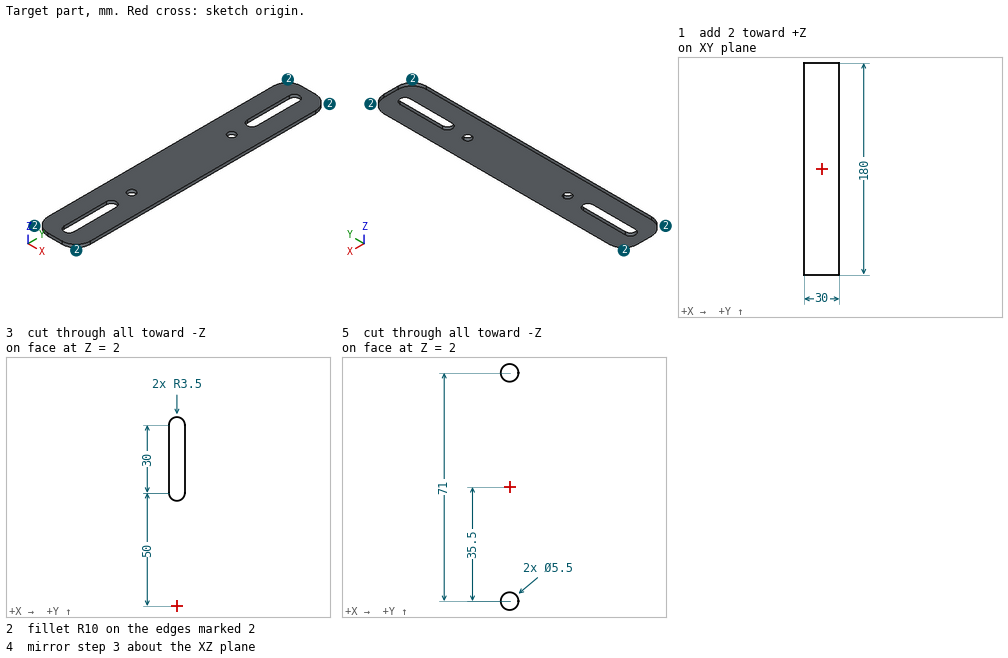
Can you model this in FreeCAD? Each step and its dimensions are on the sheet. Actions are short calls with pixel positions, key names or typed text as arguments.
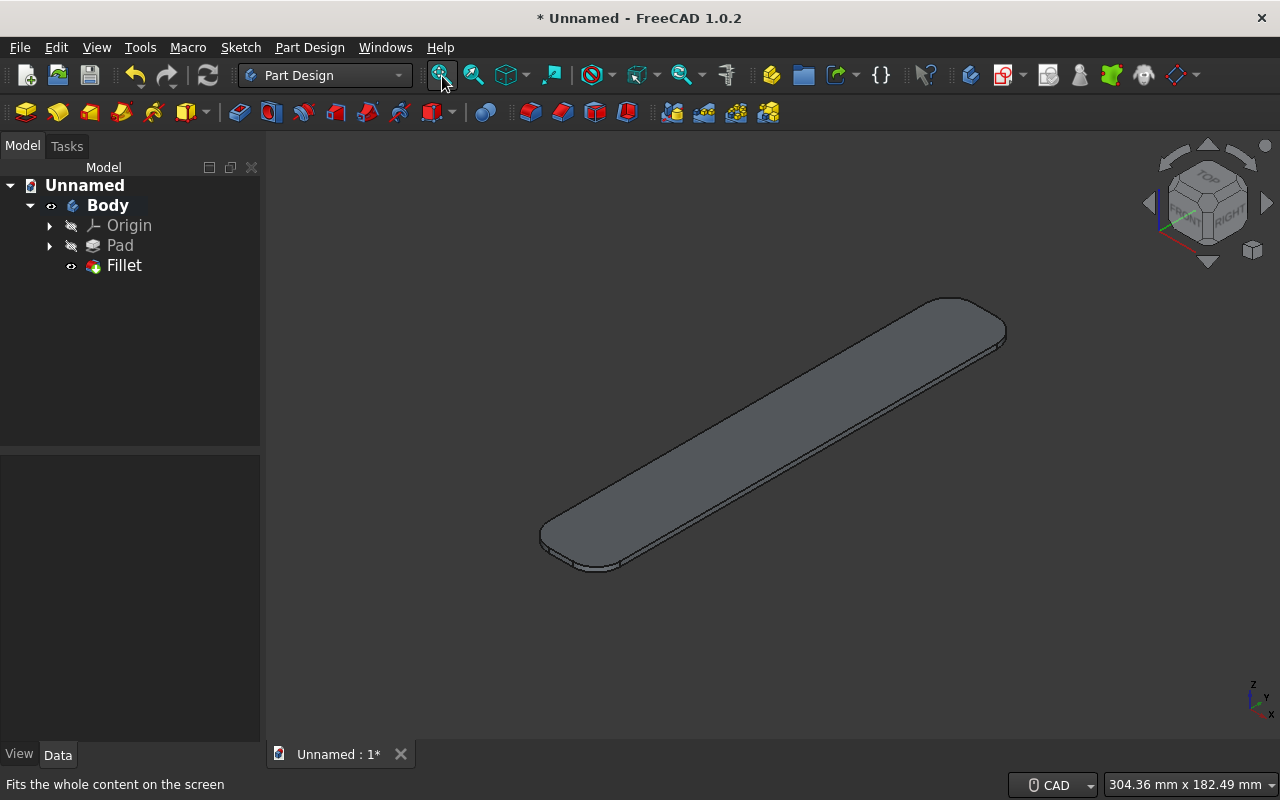
click(894, 361)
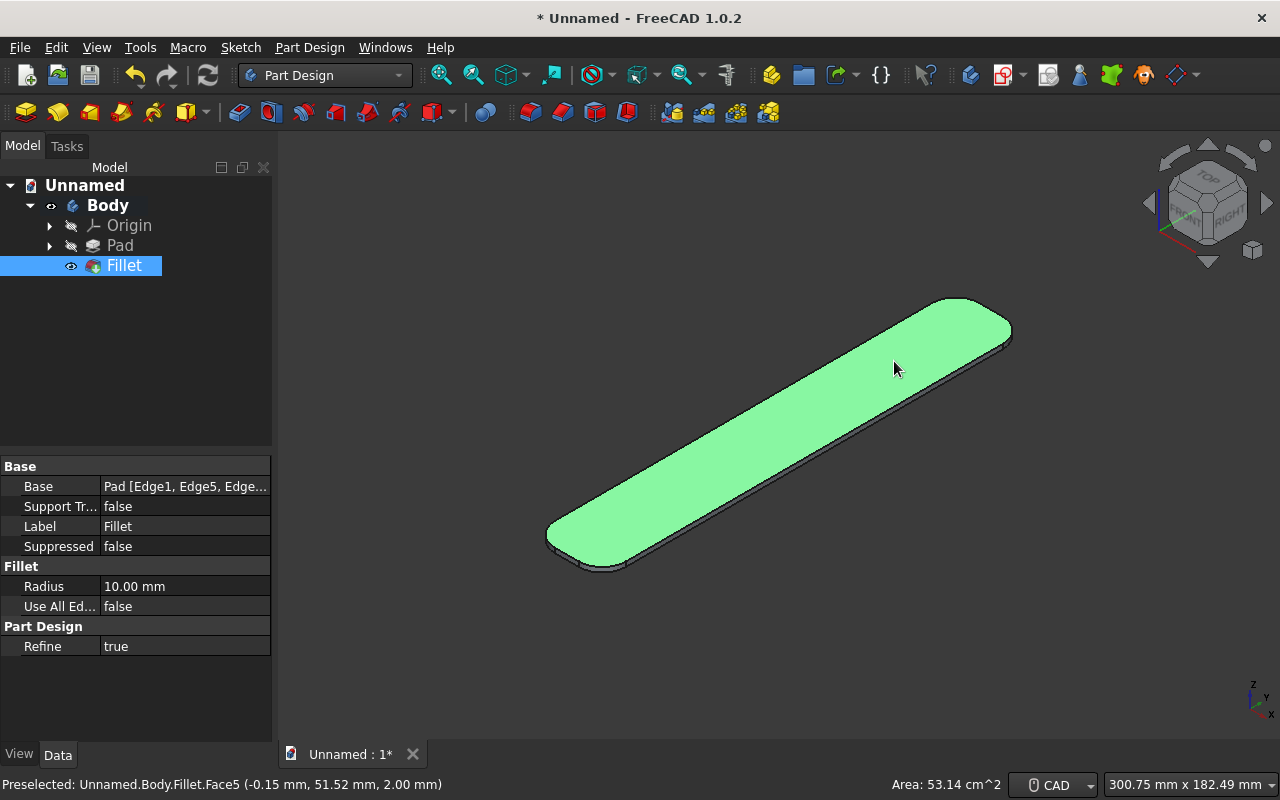
click(1004, 76)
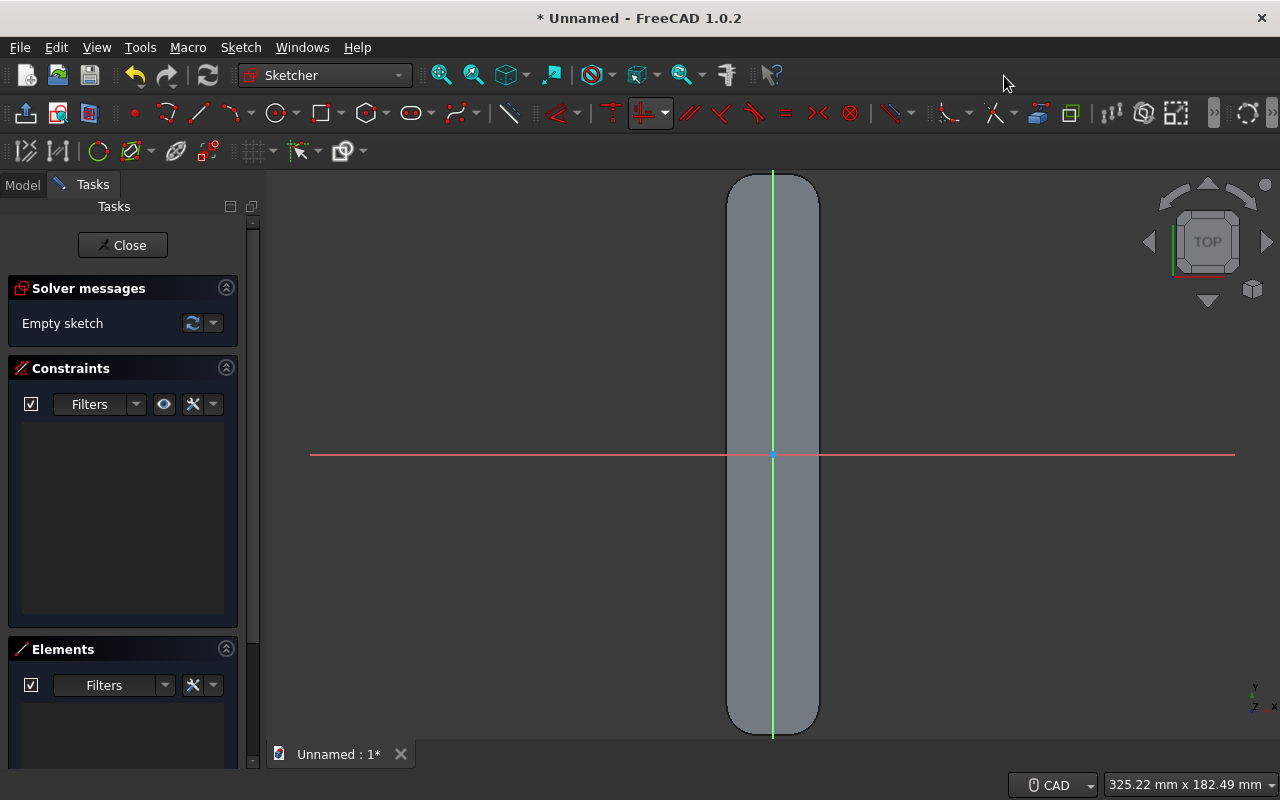
scroll(395, 711, down, 1)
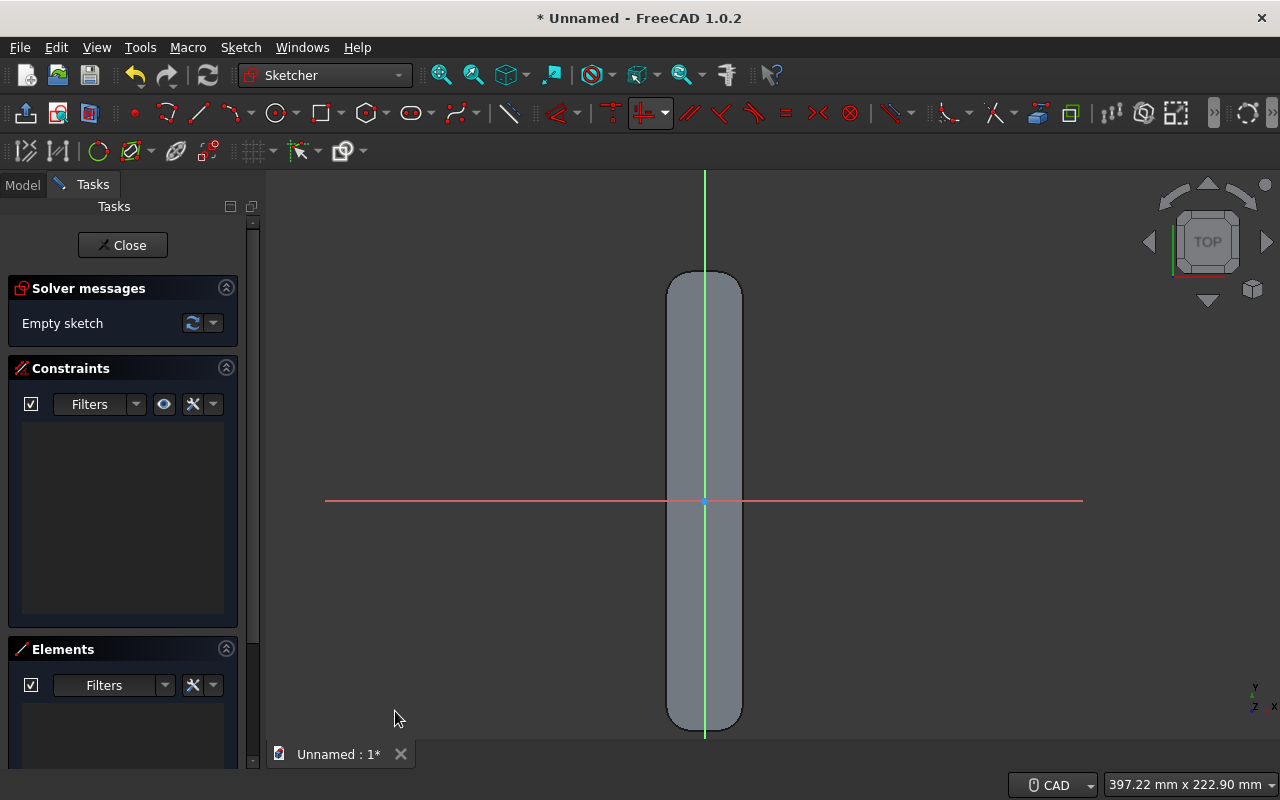
scroll(705, 322, up, 3)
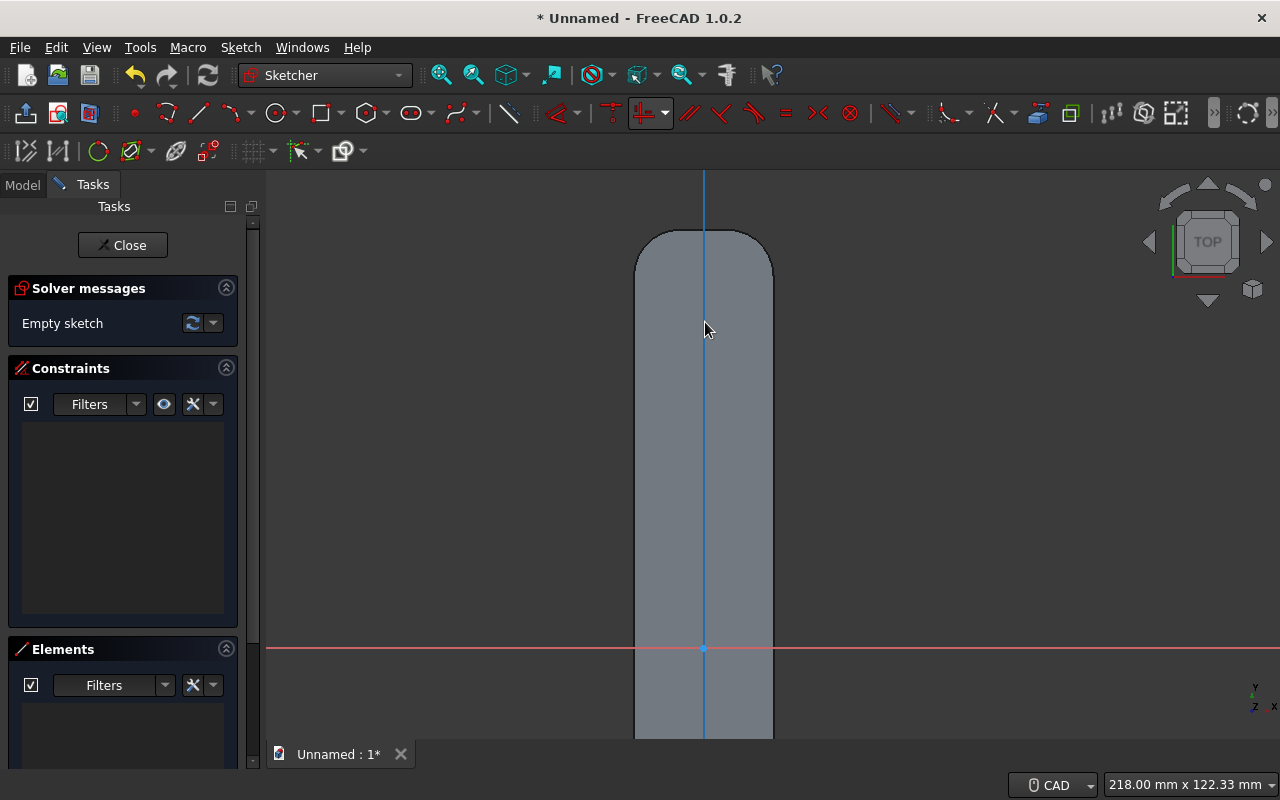
key(g)
key(s)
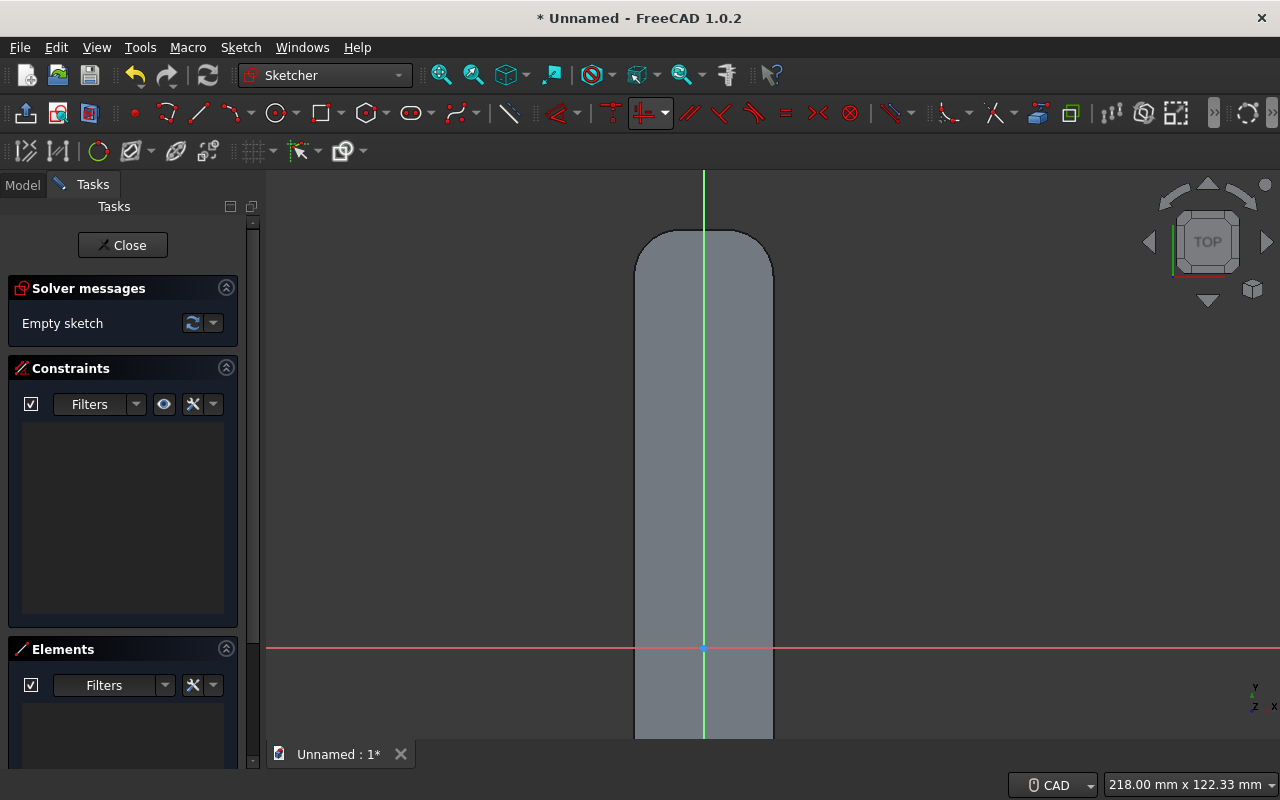
scroll(704, 416, up, 2)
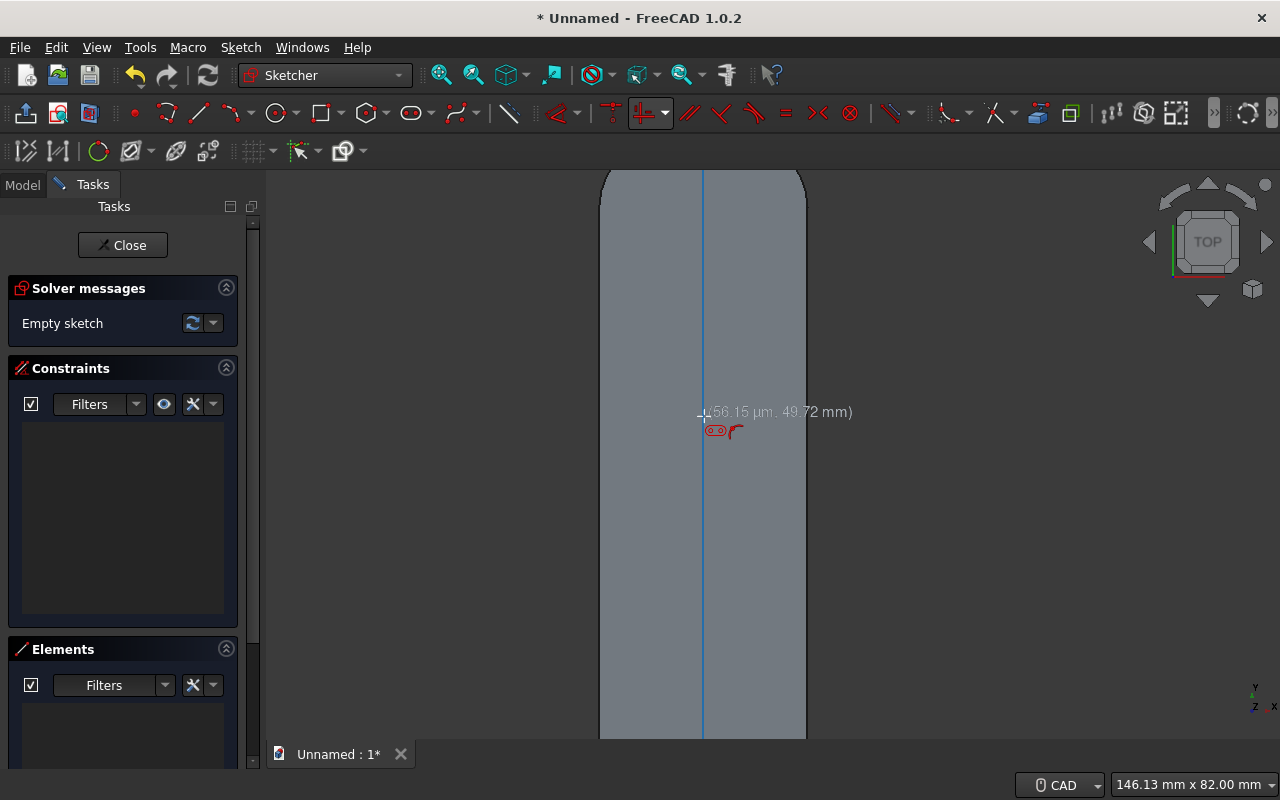
click(703, 415)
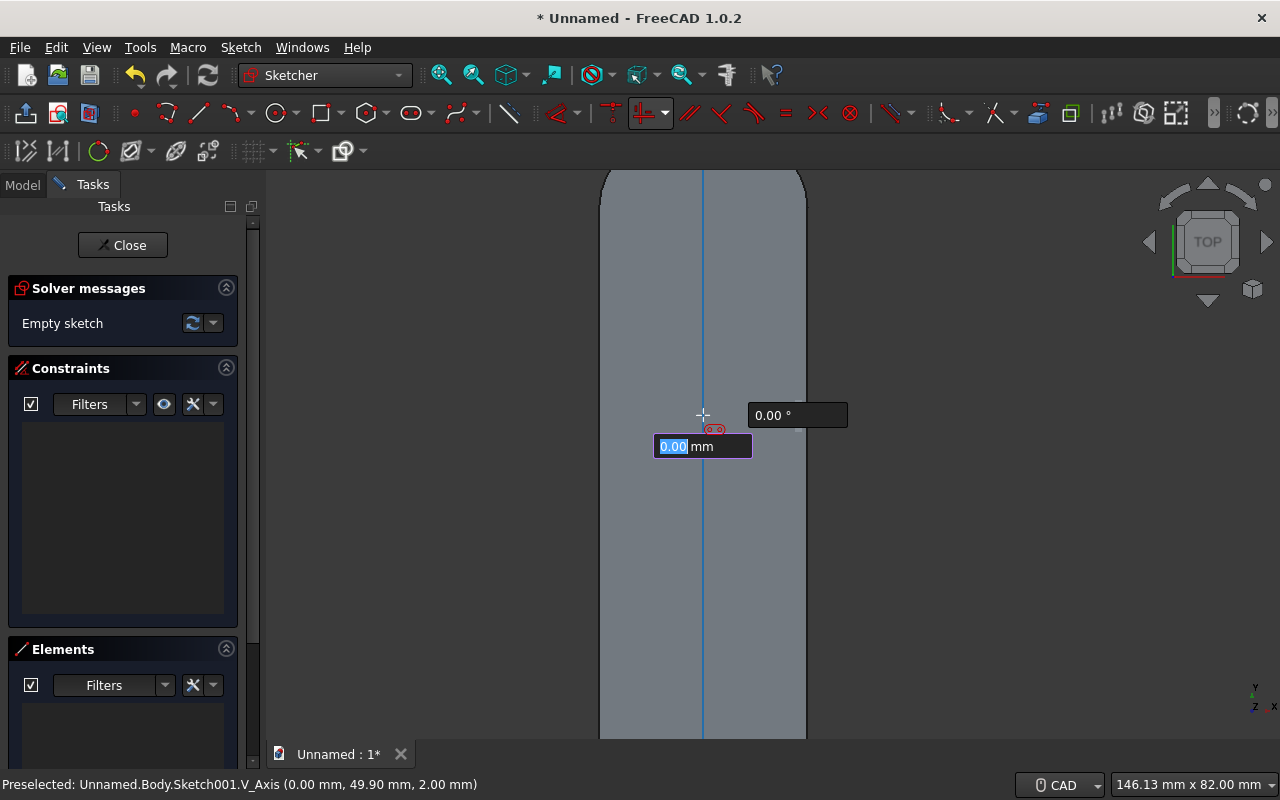
click(712, 207)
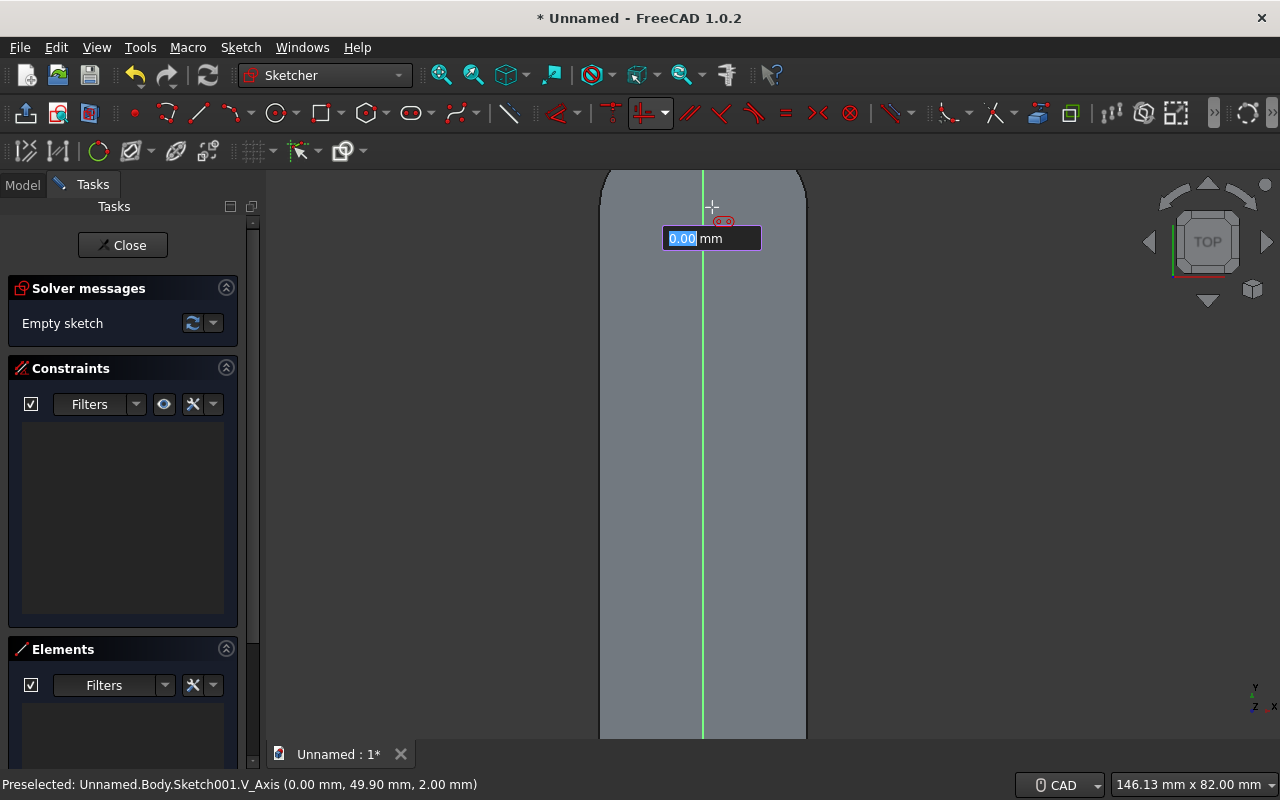
click(728, 311)
key(Escape)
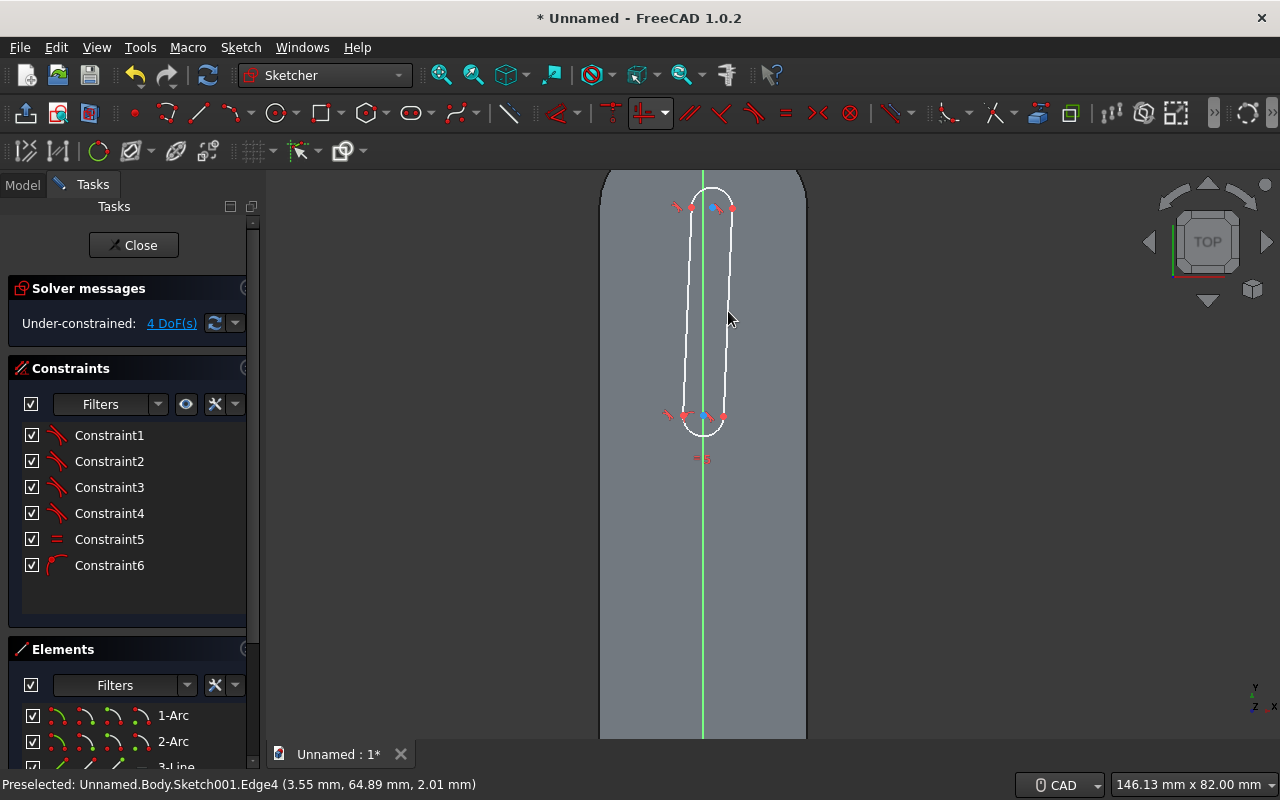
click(686, 353)